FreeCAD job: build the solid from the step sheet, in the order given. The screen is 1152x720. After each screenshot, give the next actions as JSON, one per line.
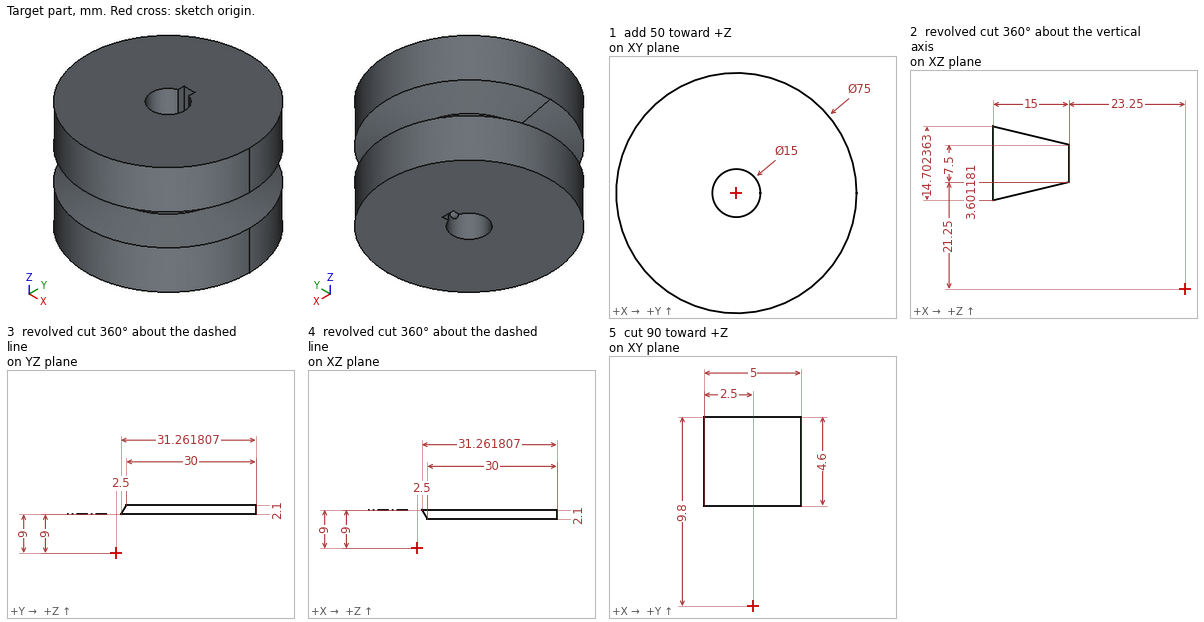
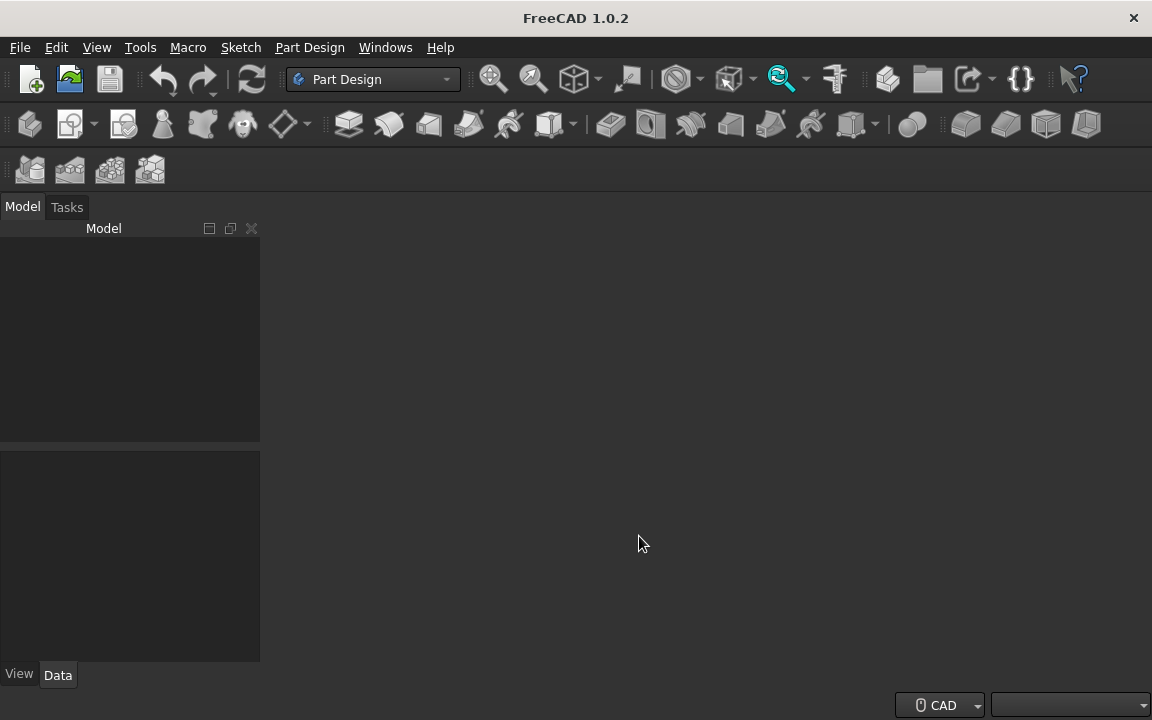
{"action": "left_click", "coordinate": [30, 80]}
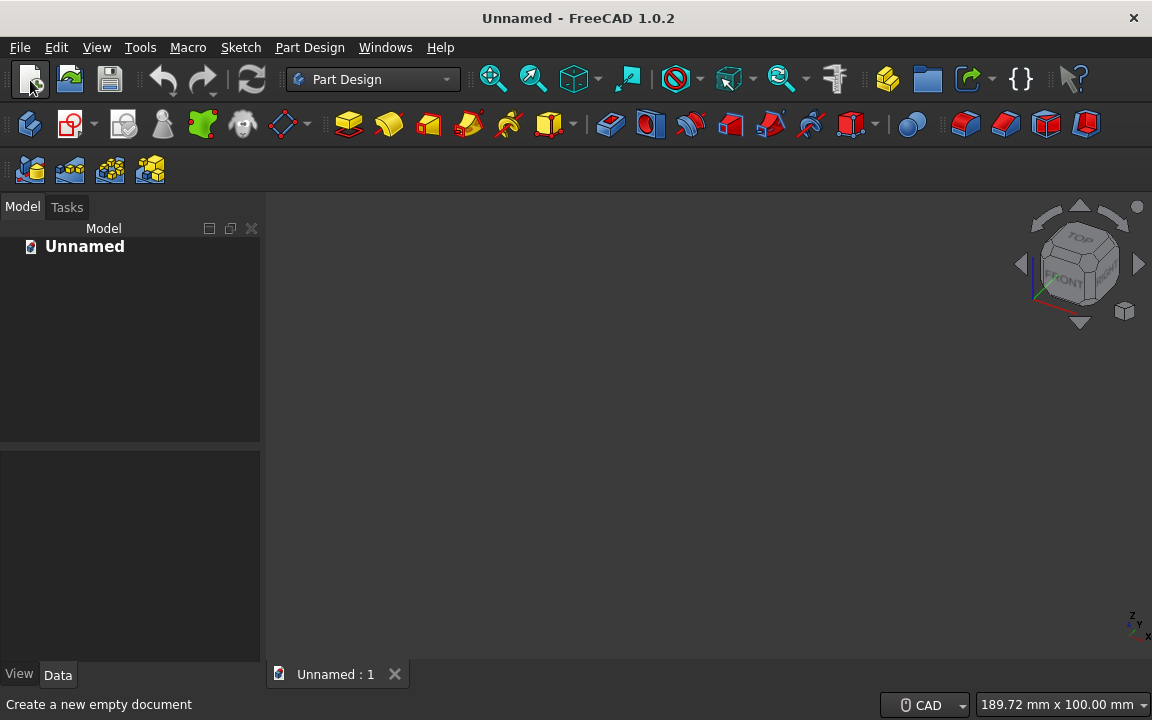
{"action": "left_click", "coordinate": [70, 124]}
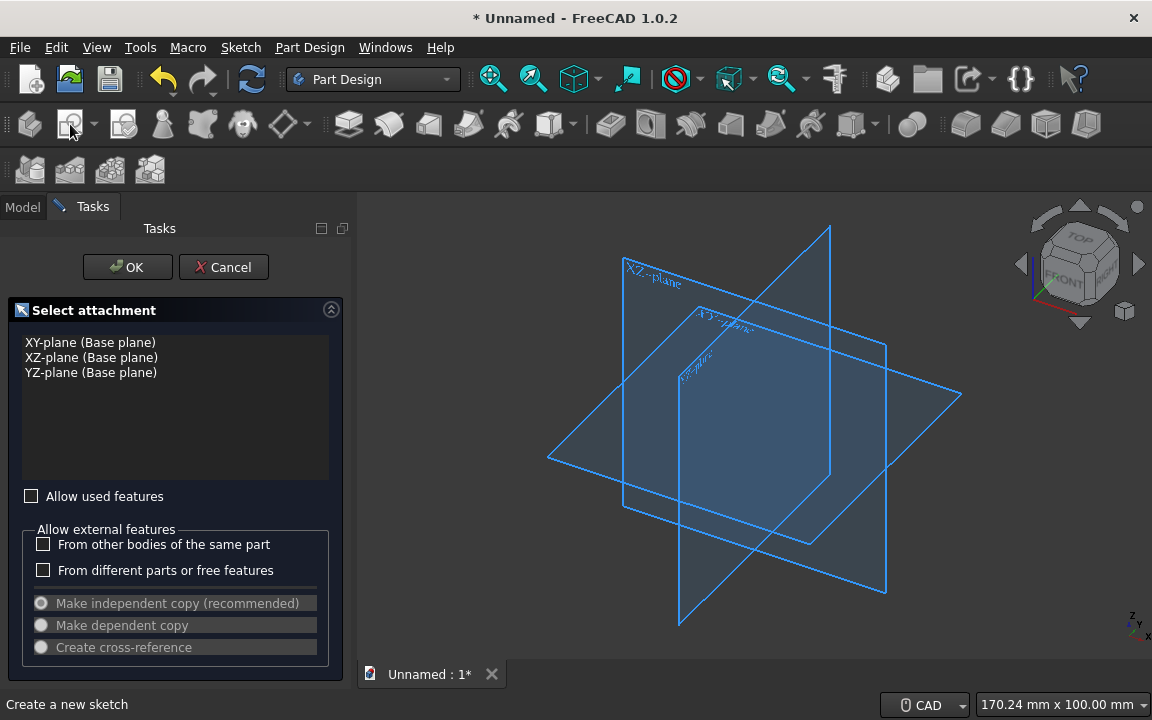
{"action": "left_click", "coordinate": [82, 342]}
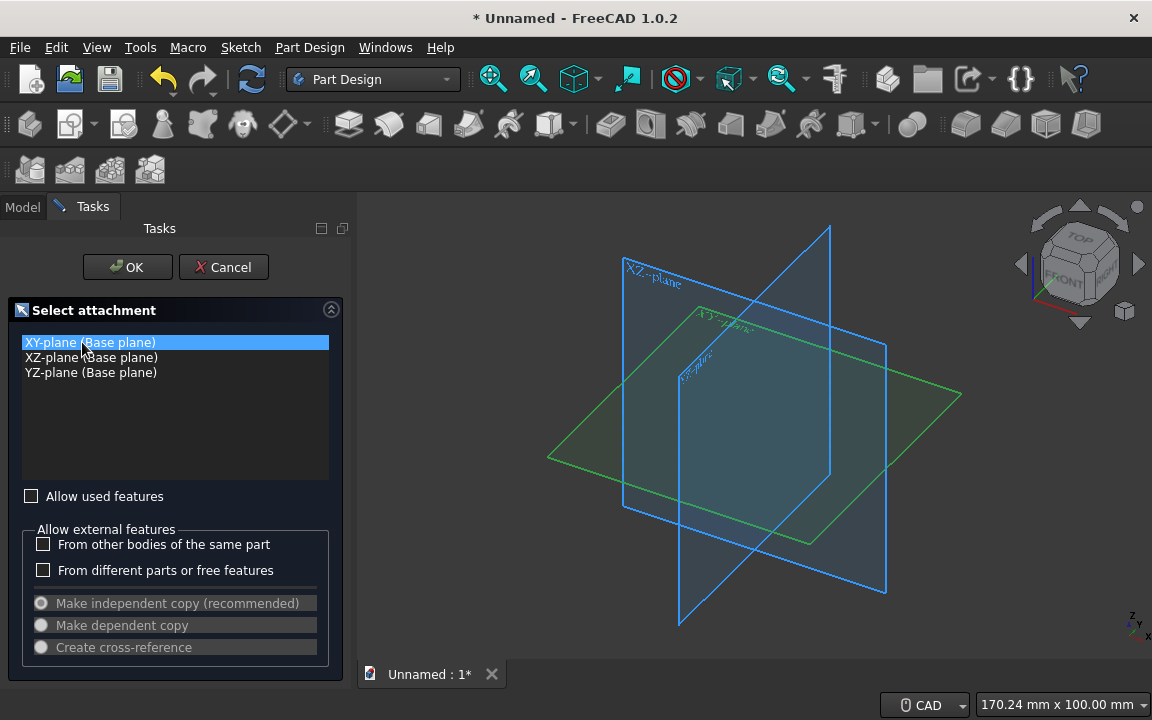
{"action": "left_click", "coordinate": [128, 267]}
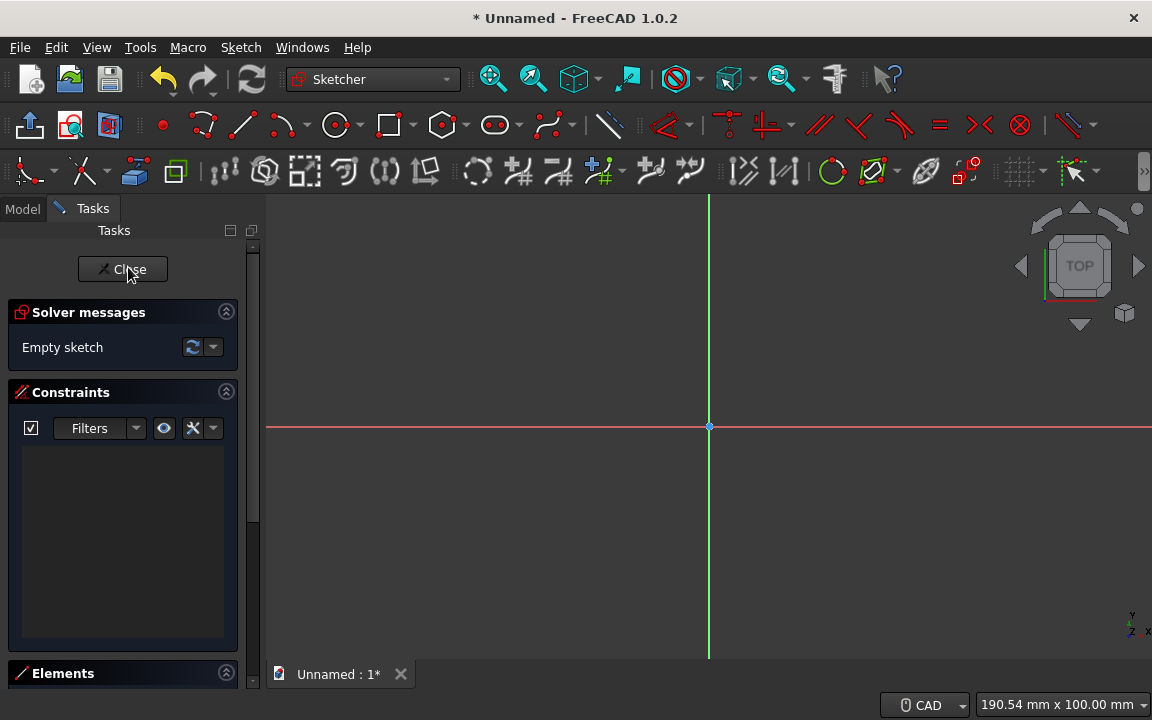
{"action": "left_click", "coordinate": [336, 126]}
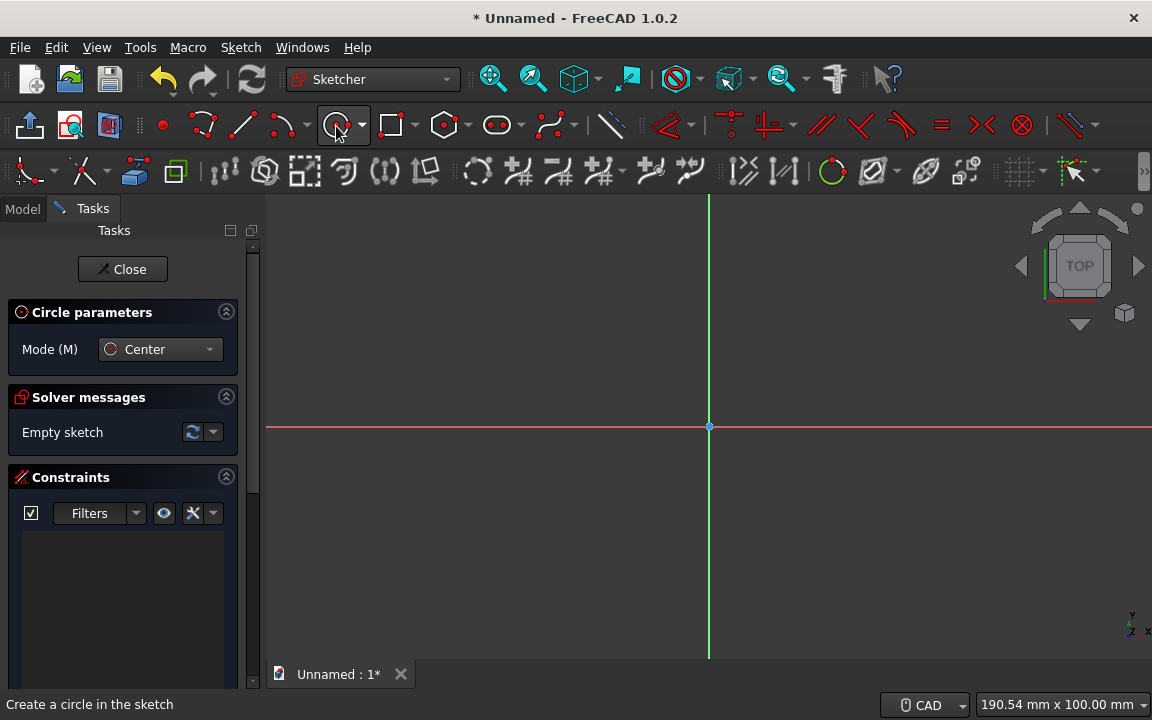
{"action": "left_click", "coordinate": [709, 426]}
{"action": "mouse_move", "coordinate": [832, 303]}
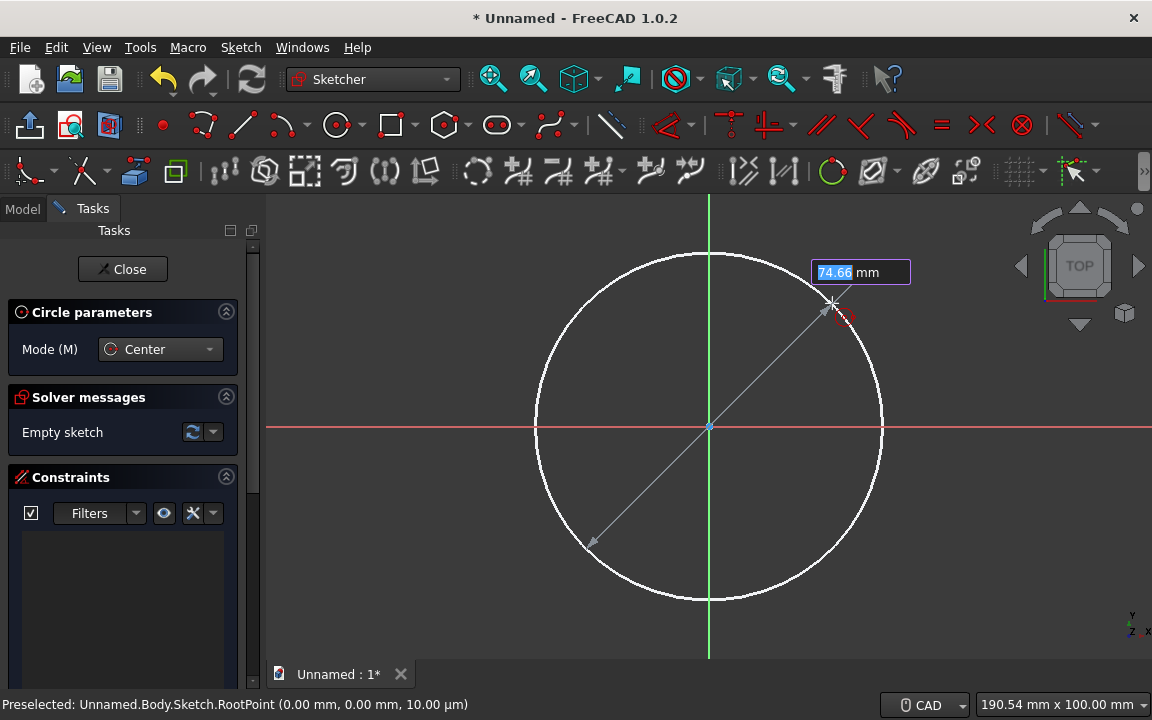
{"action": "type", "text": "75"}
{"action": "key", "text": "Return"}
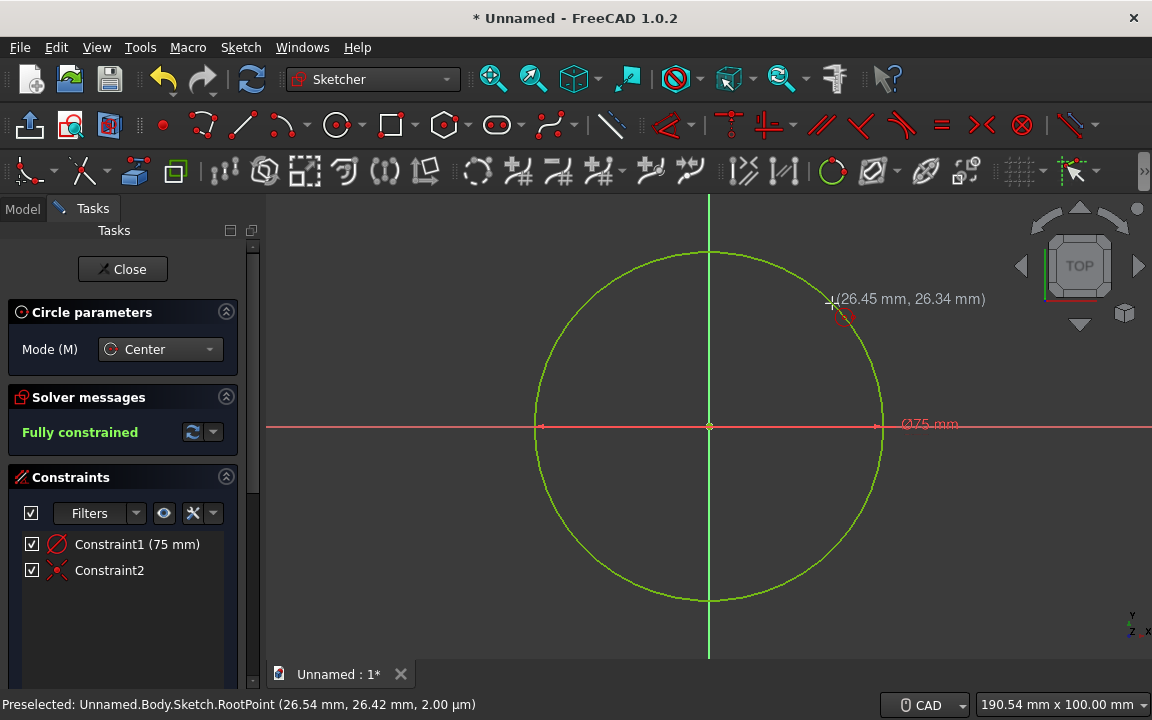
{"action": "left_click", "coordinate": [709, 426]}
{"action": "mouse_move", "coordinate": [734, 402]}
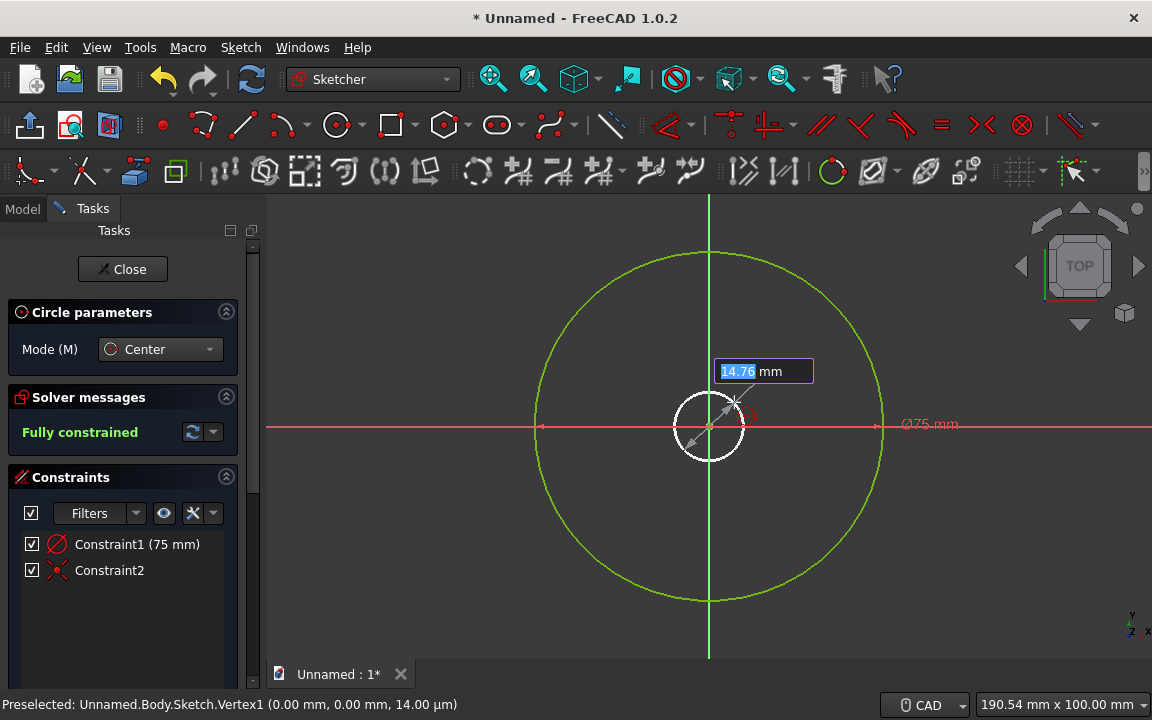
{"action": "type", "text": "15"}
{"action": "key", "text": "Return"}
{"action": "key", "text": "Escape"}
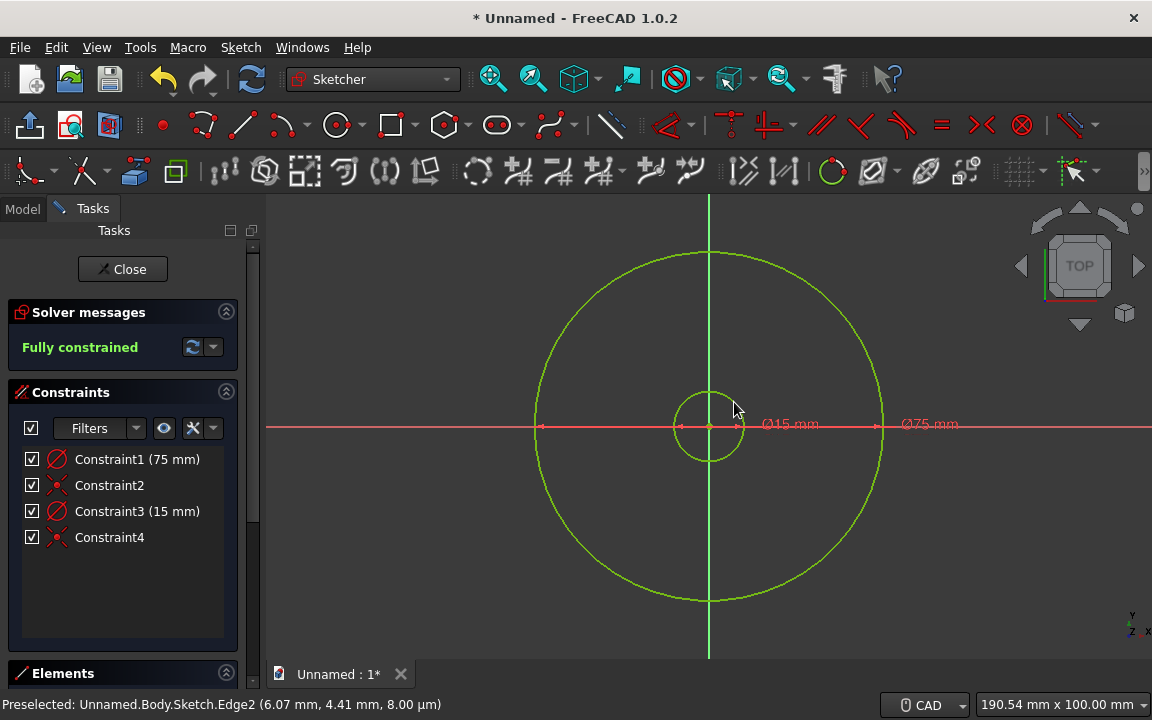
{"action": "left_click", "coordinate": [123, 269]}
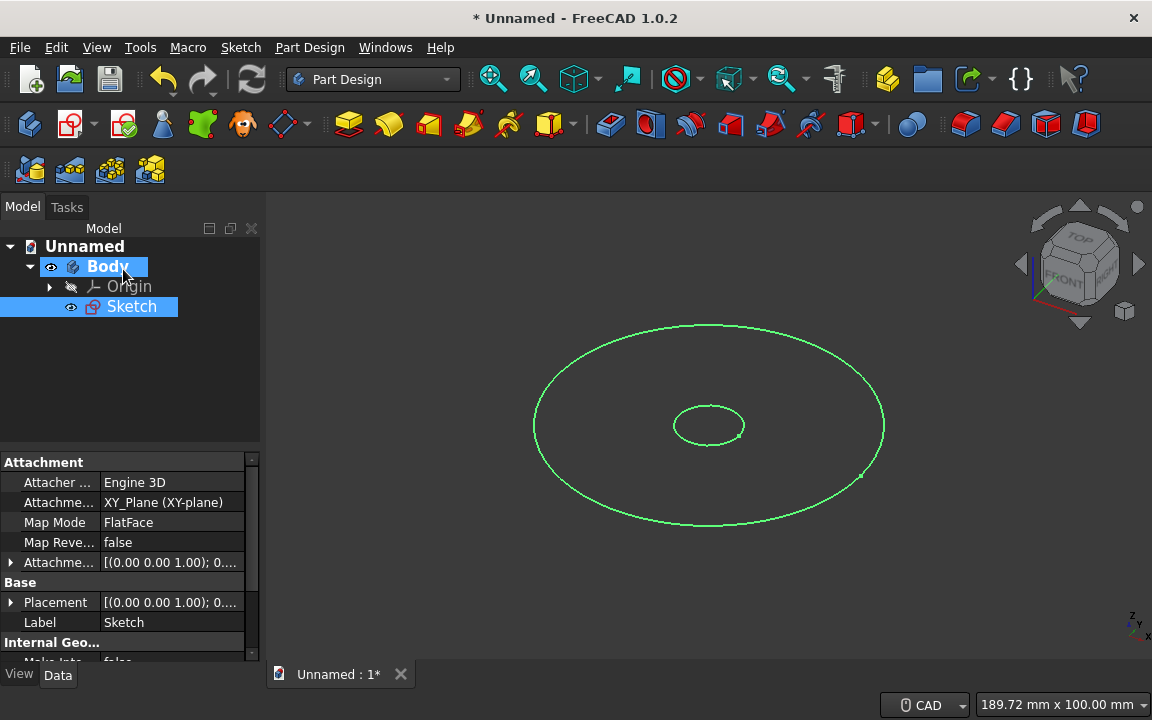
{"action": "left_click", "coordinate": [350, 124]}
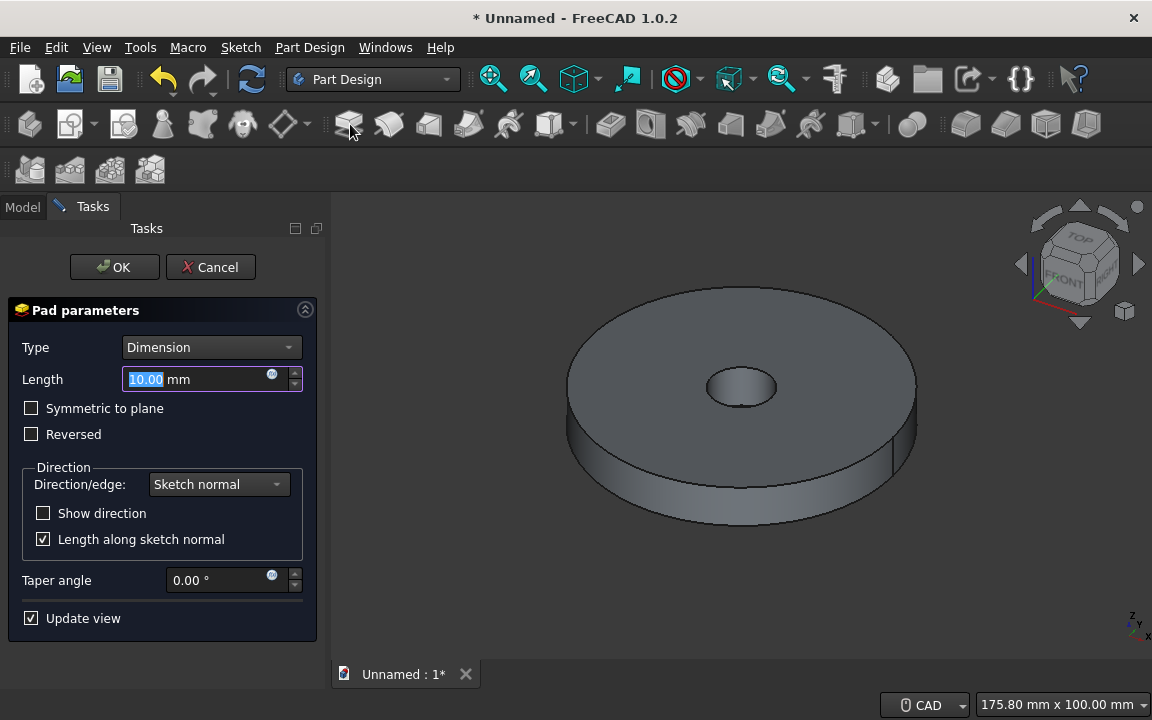
{"action": "type", "text": "50"}
{"action": "key", "text": "Tab"}